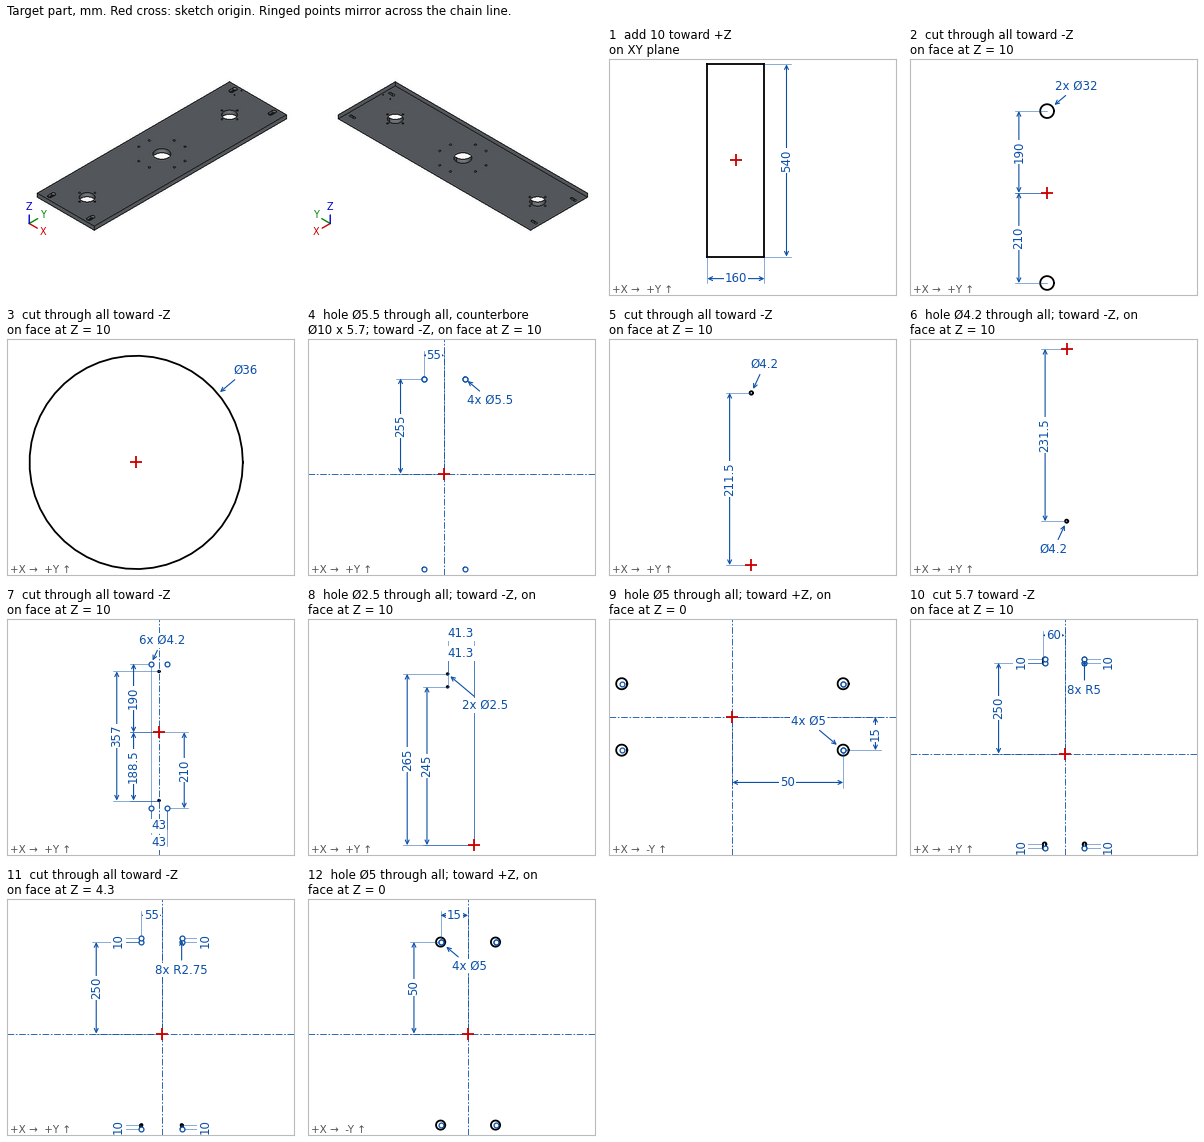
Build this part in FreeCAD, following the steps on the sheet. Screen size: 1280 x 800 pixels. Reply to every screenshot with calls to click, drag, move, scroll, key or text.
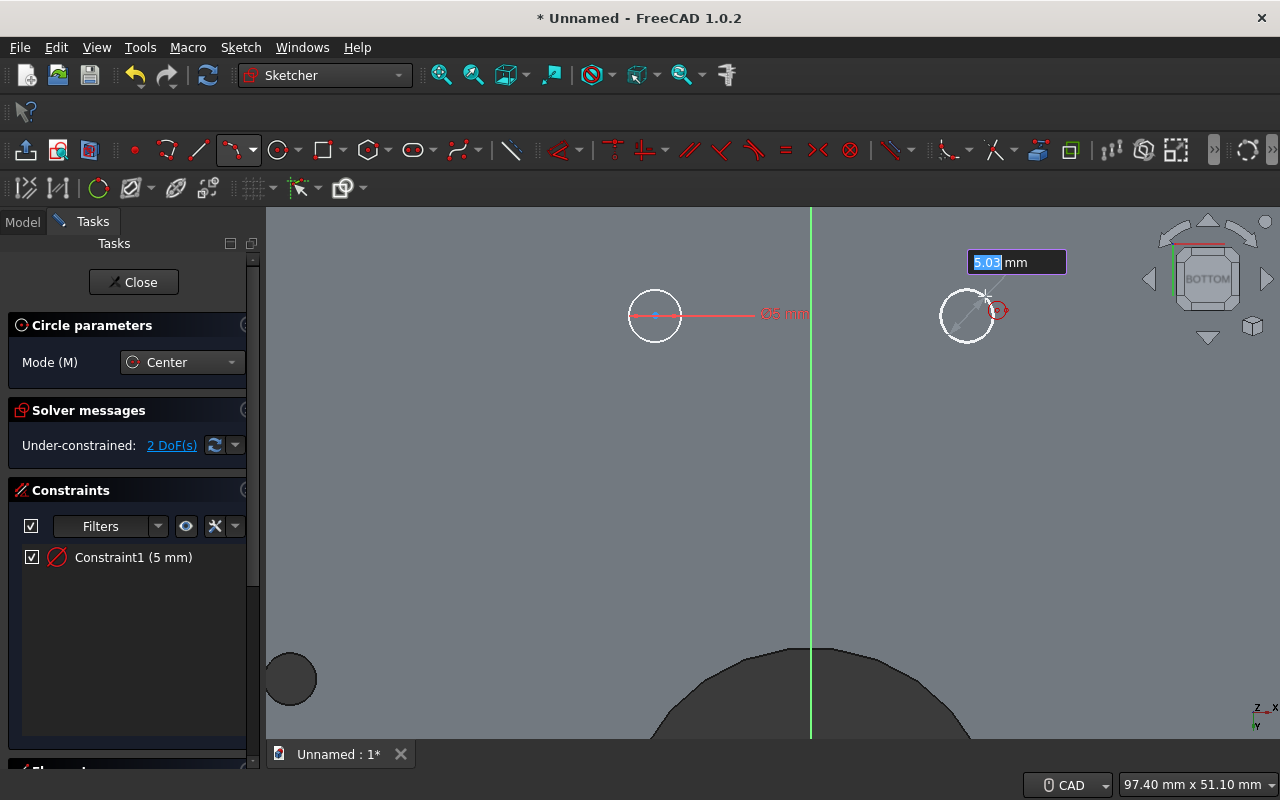
text(5)
key(Return)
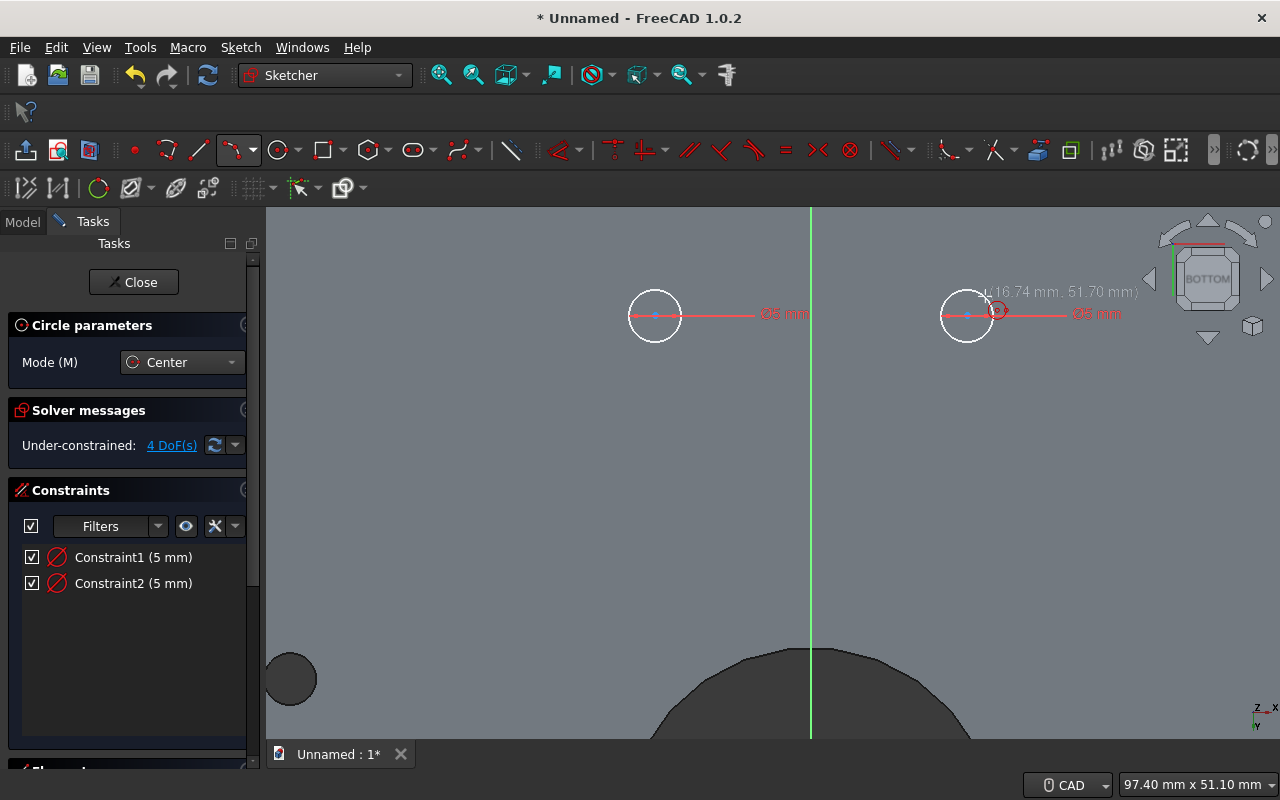
scroll(659, 317, down, 6)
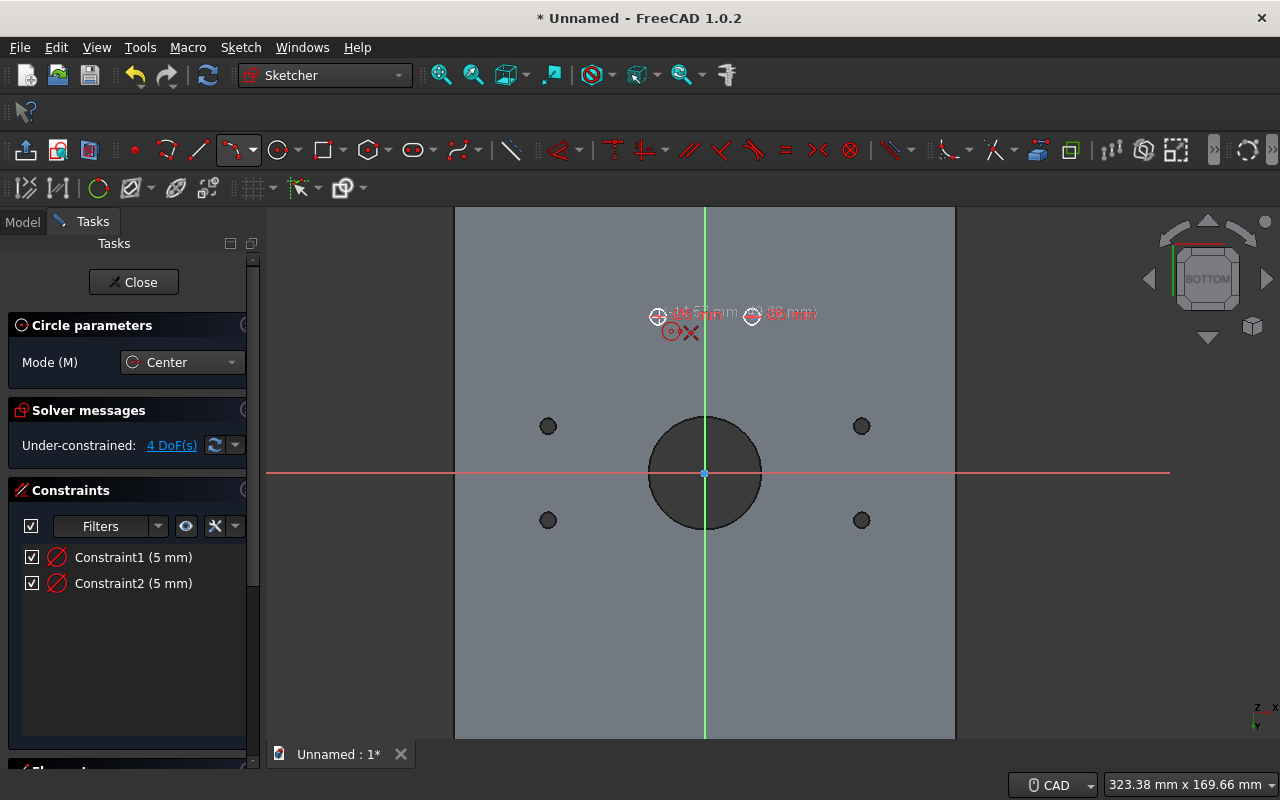
scroll(752, 630, up, 6)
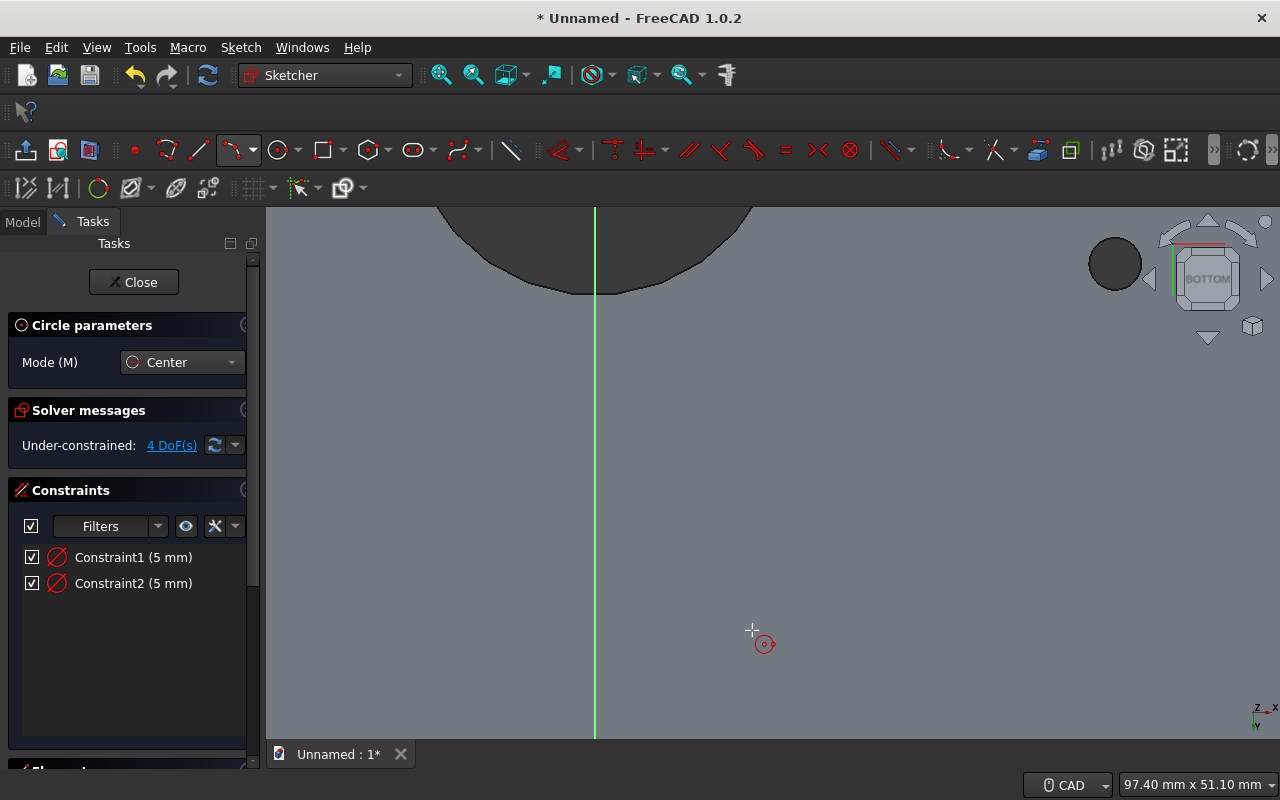
click(751, 628)
move(769, 610)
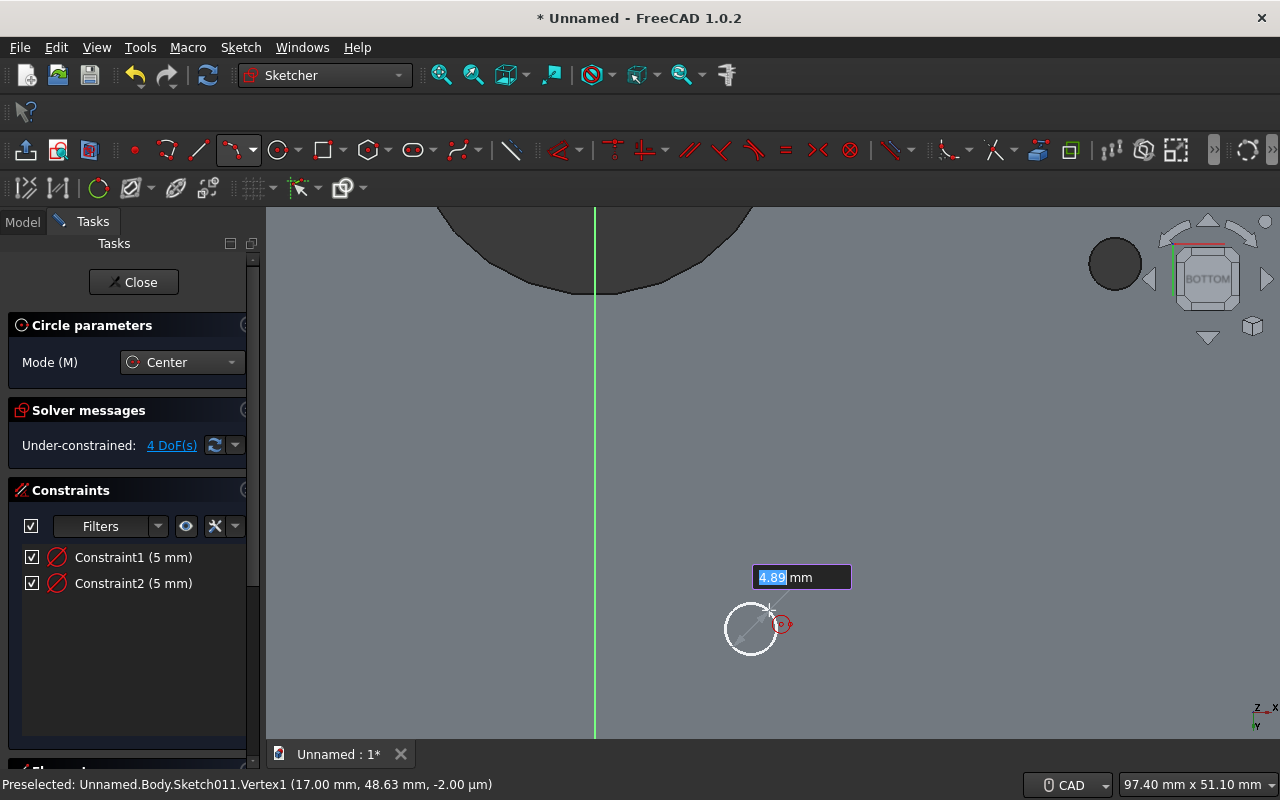
text(5)
key(Return)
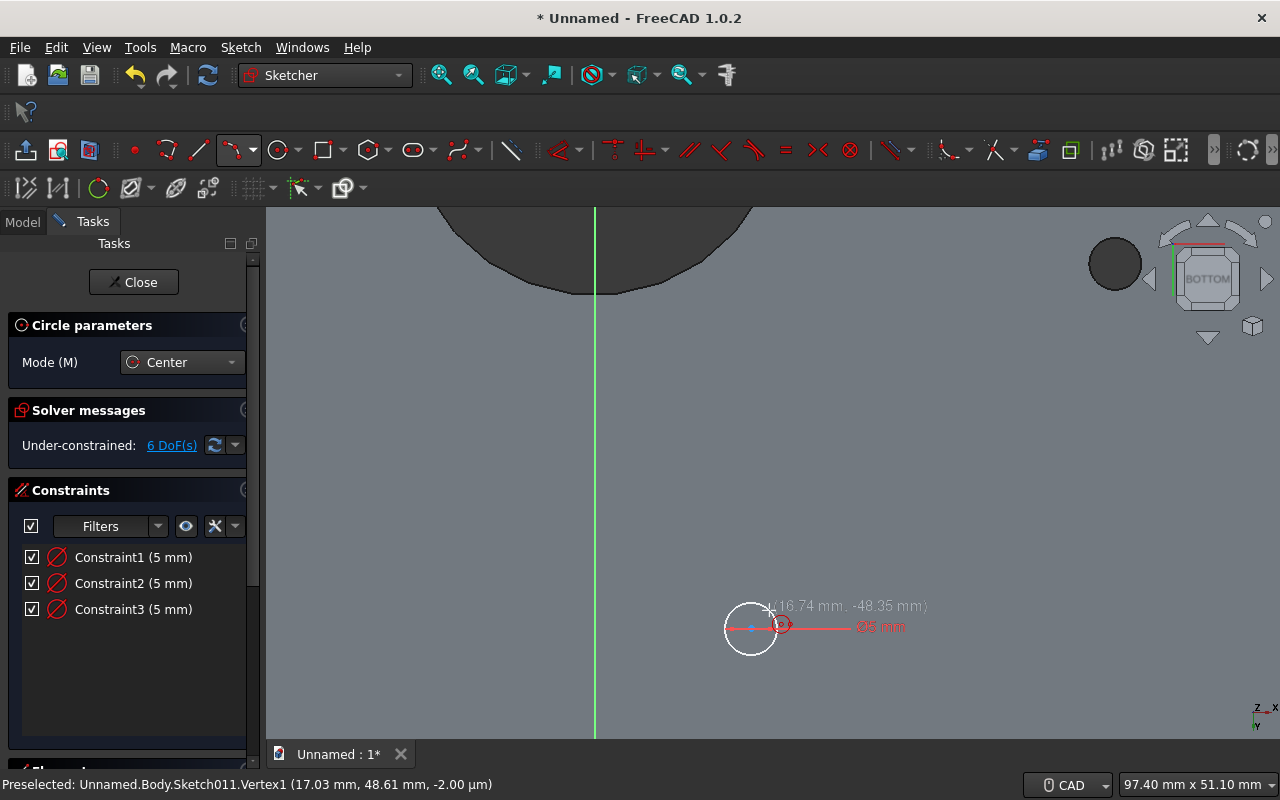
click(439, 628)
move(457, 610)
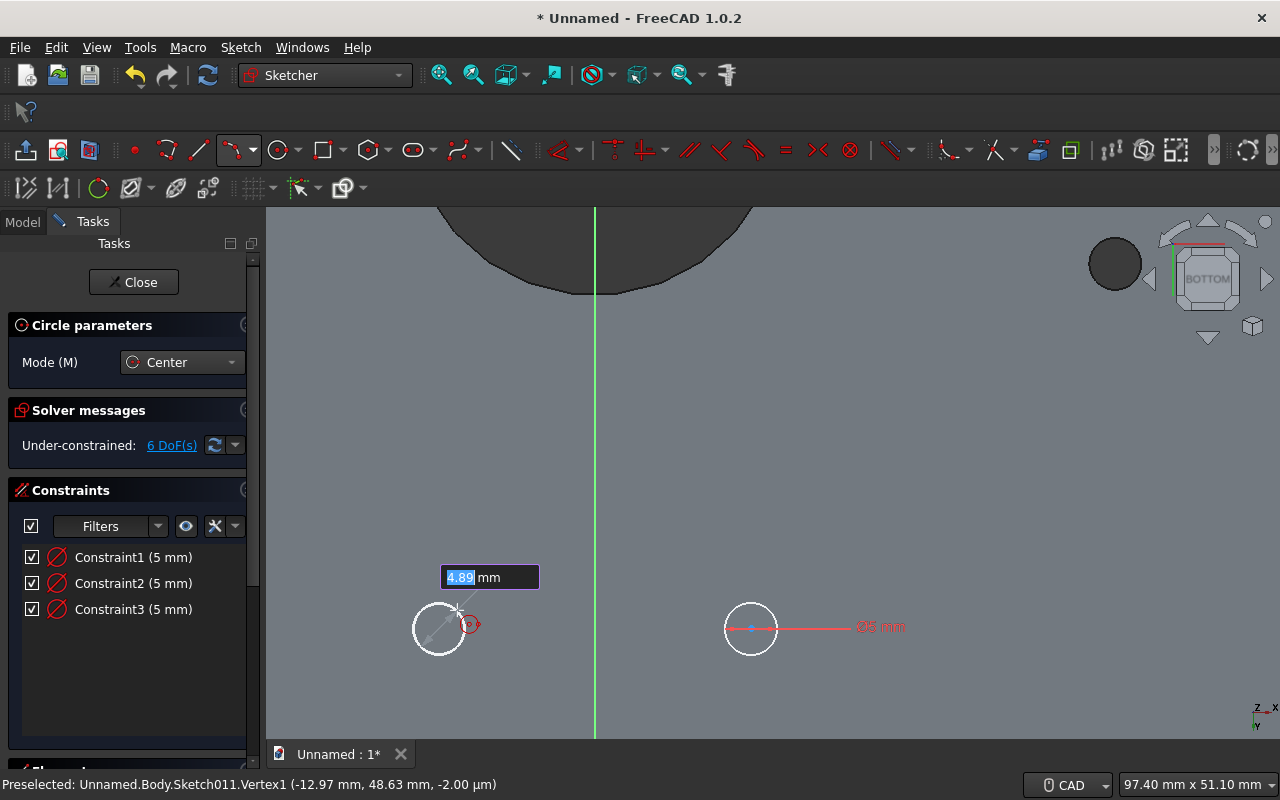
text(5)
key(Return)
key(Escape)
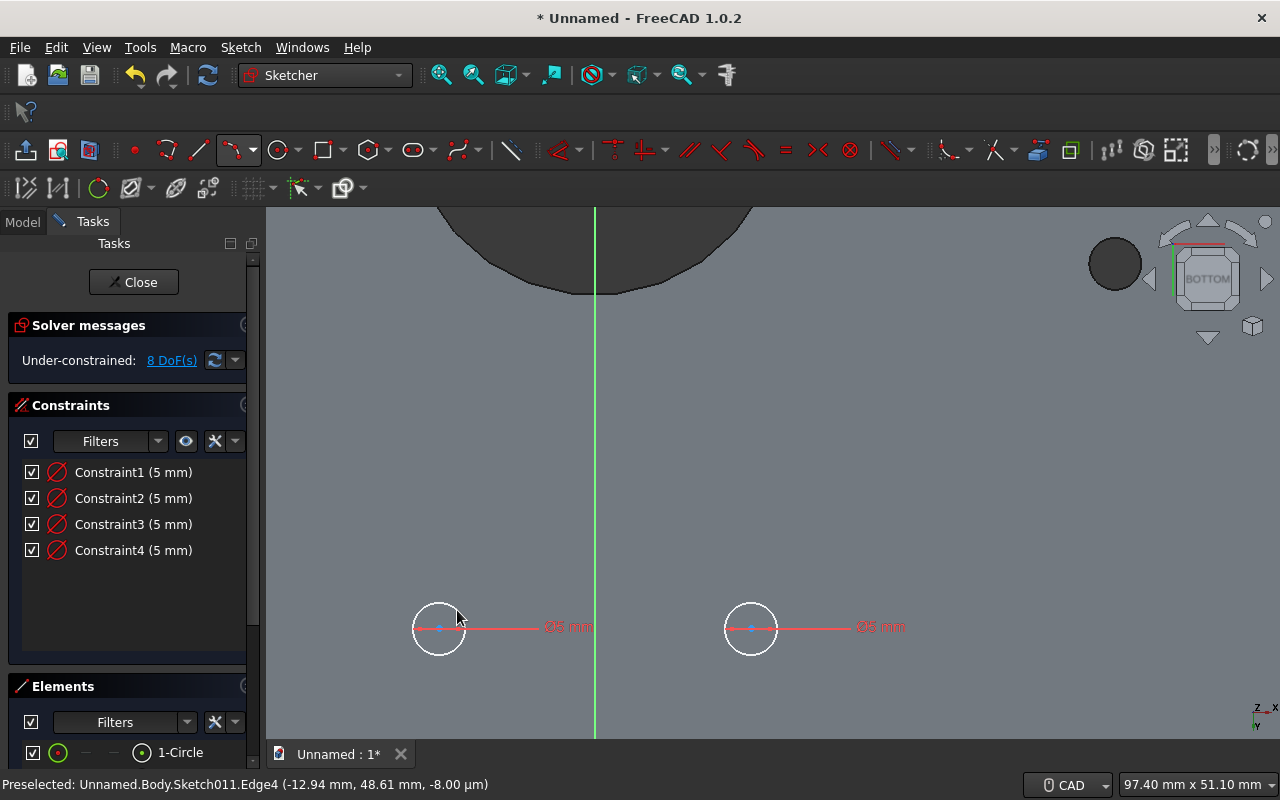
scroll(752, 630, down, 6)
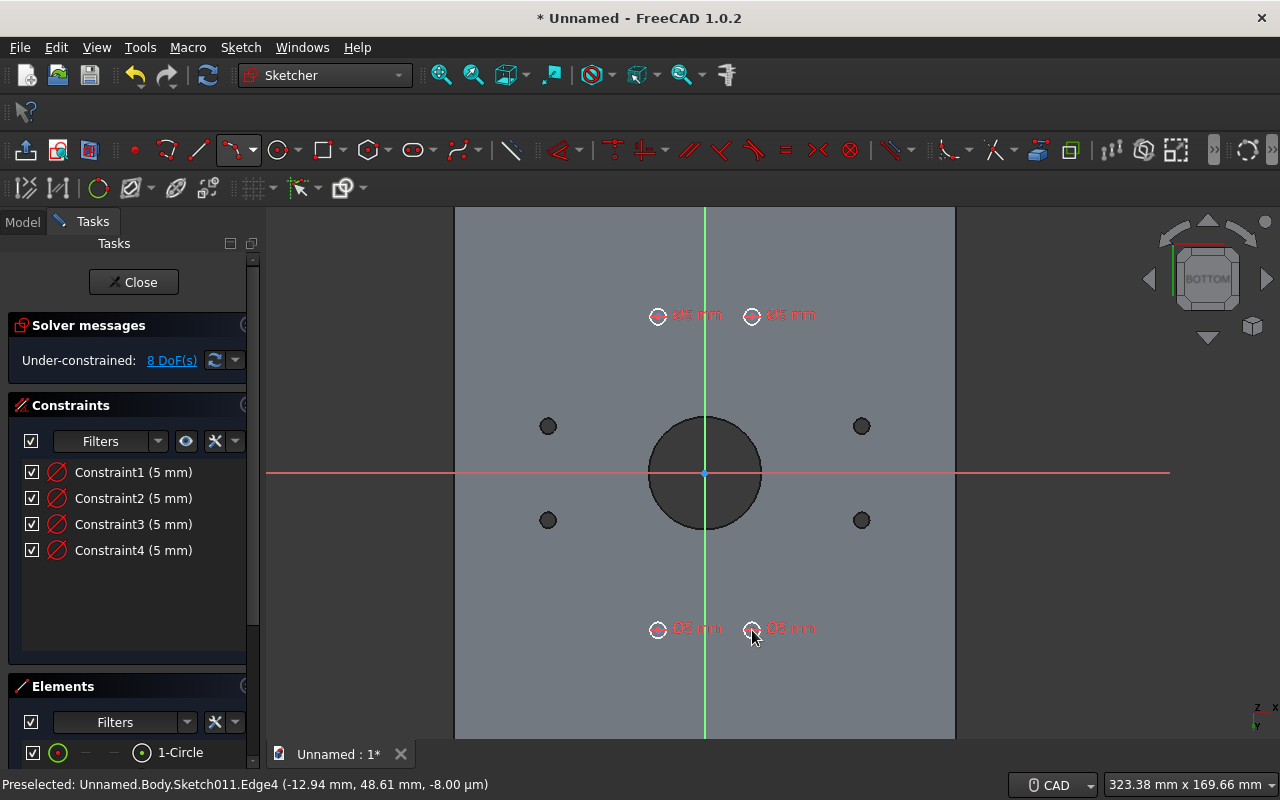
click(658, 317)